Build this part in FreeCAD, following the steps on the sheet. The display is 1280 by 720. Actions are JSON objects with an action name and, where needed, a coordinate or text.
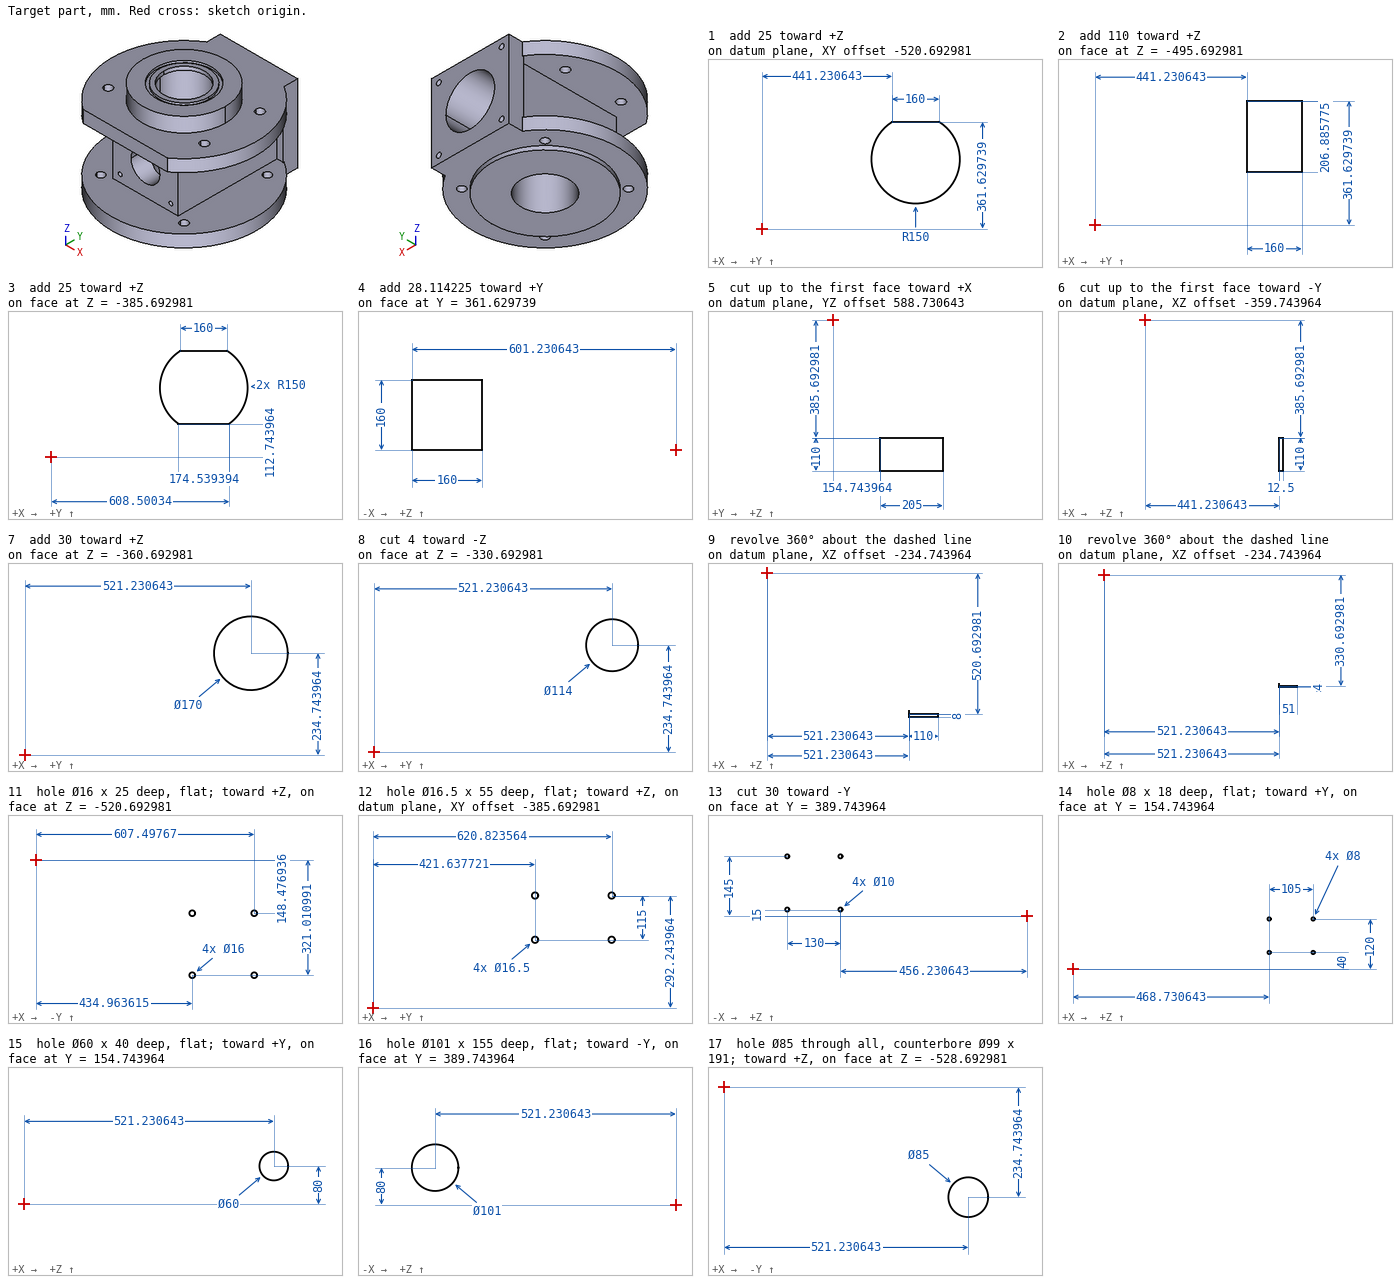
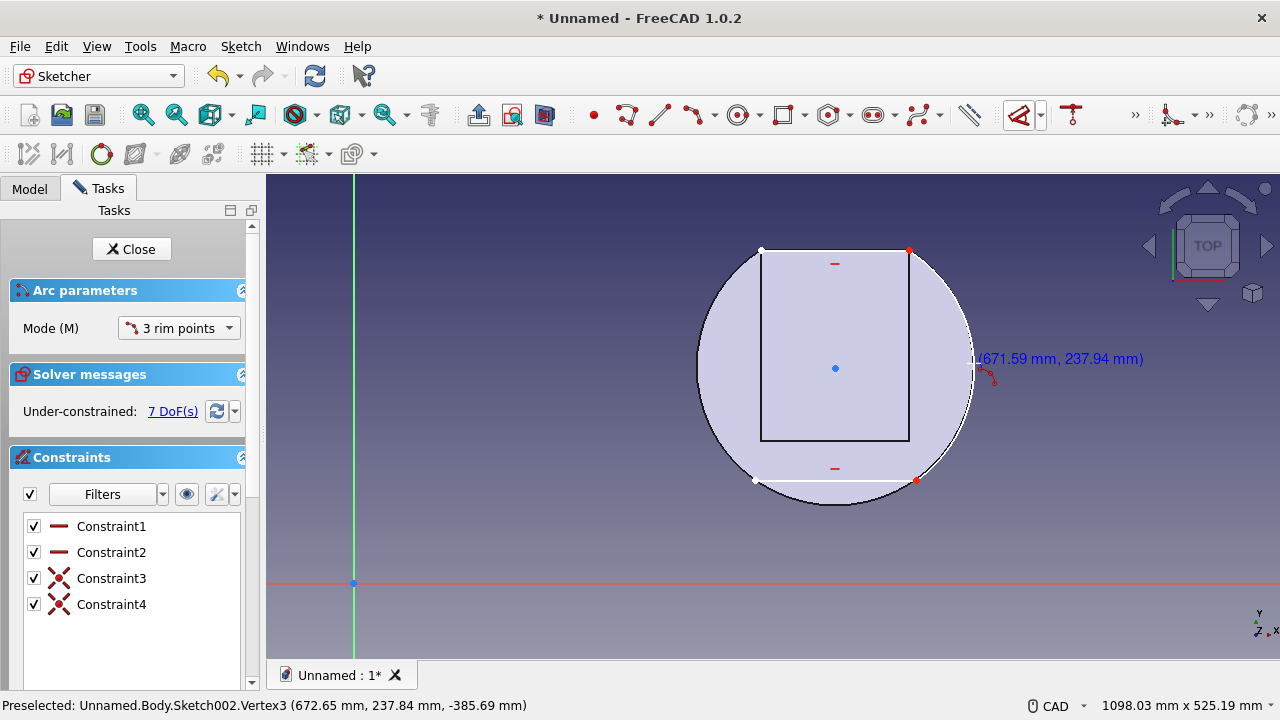
{"action": "left_click", "coordinate": [761, 251]}
{"action": "left_click", "coordinate": [755, 481]}
{"action": "left_click", "coordinate": [697, 363]}
{"action": "key", "text": "Escape"}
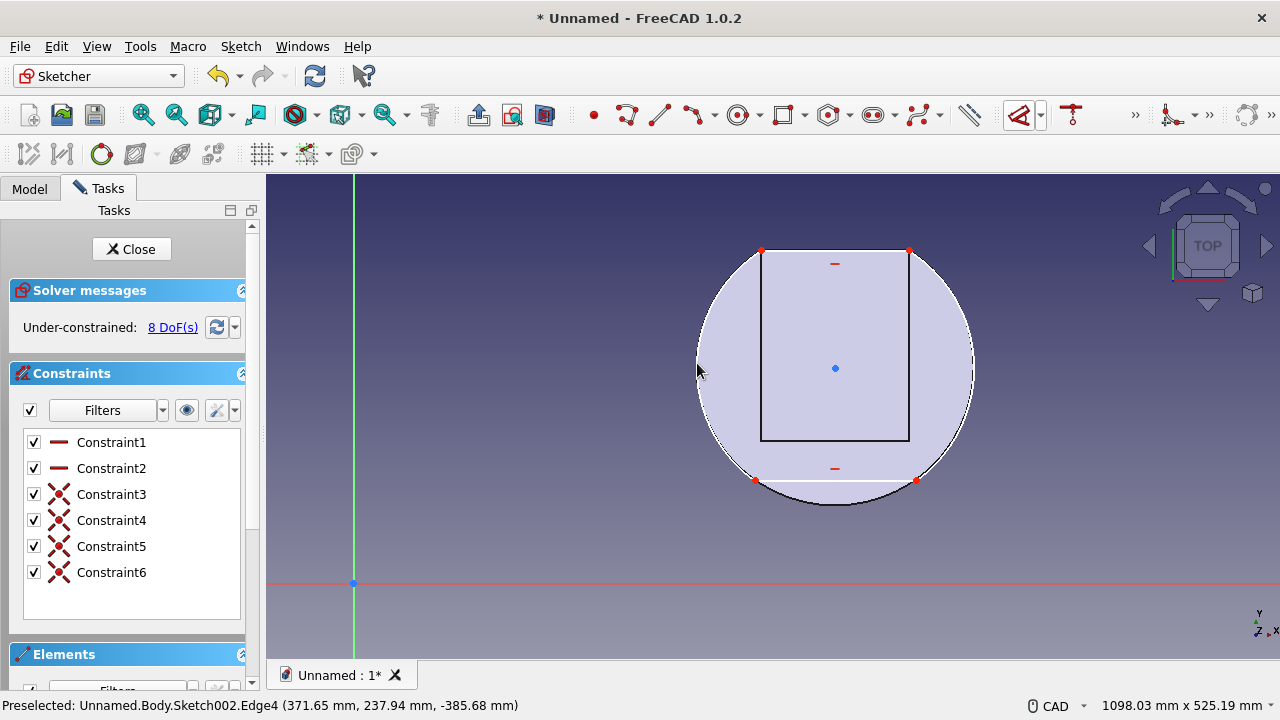
{"action": "left_click", "coordinate": [965, 417]}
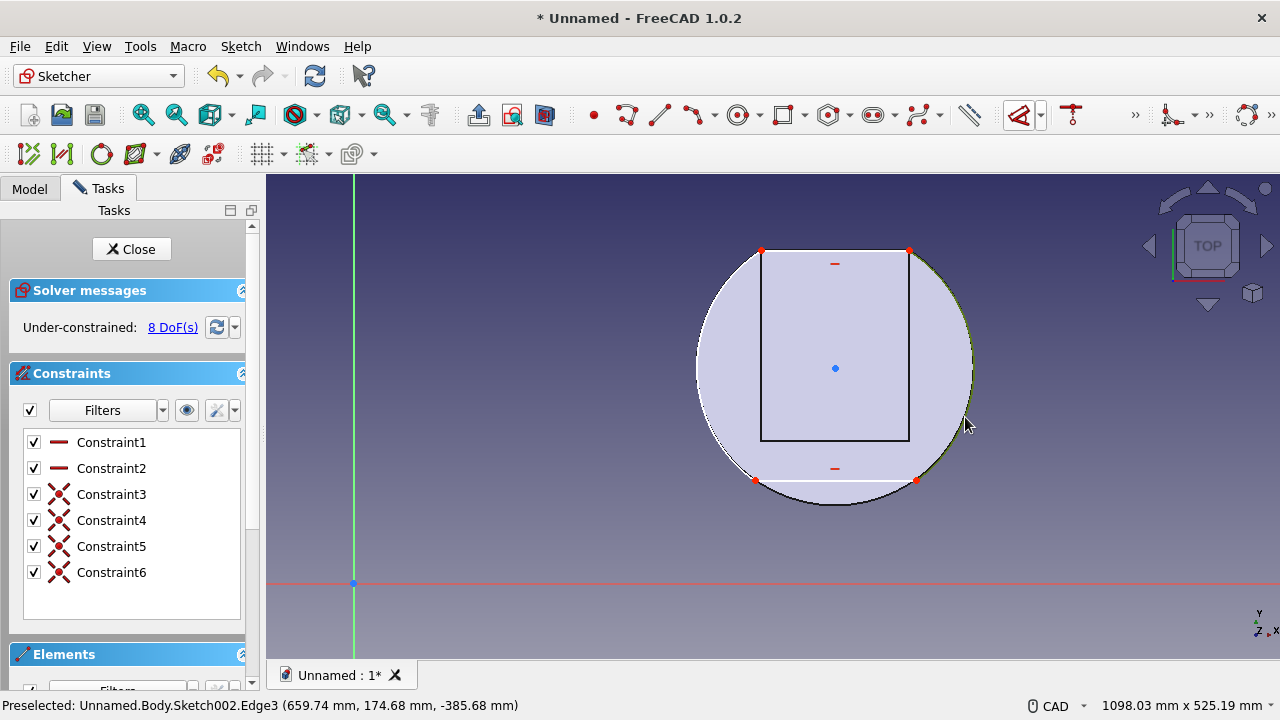
{"action": "left_click", "coordinate": [709, 312]}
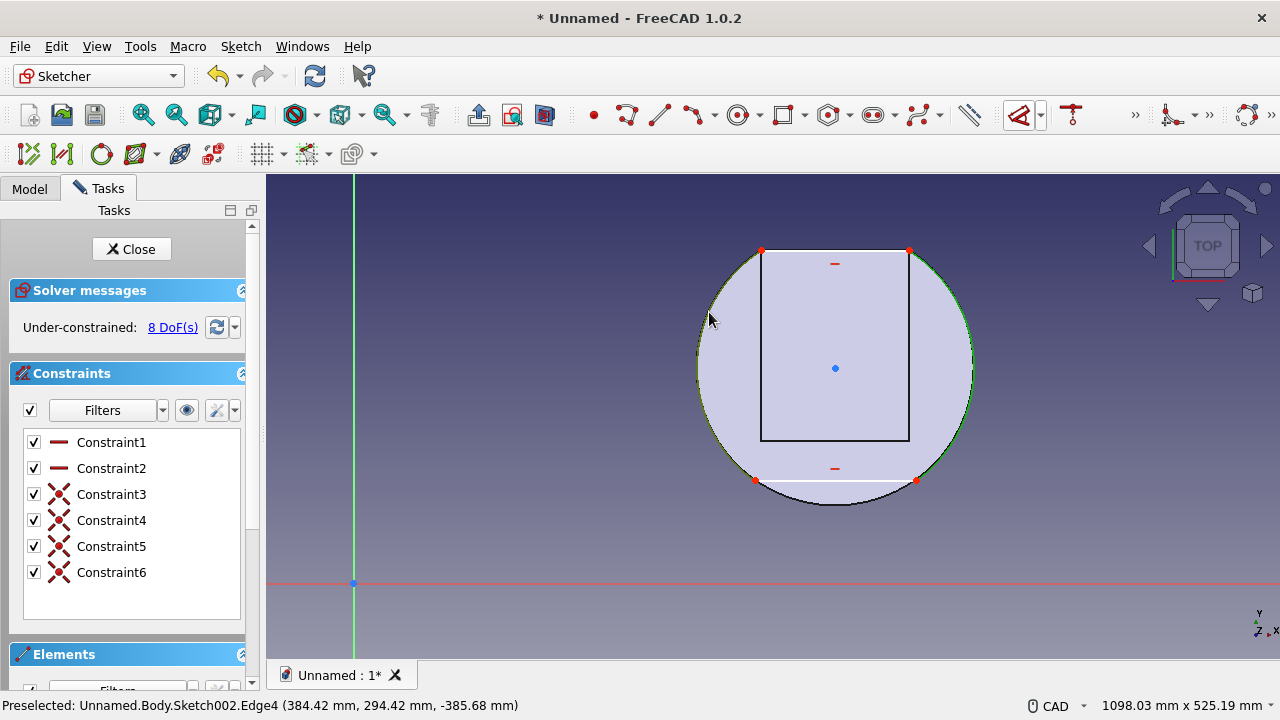
{"action": "left_click", "coordinate": [1071, 116]}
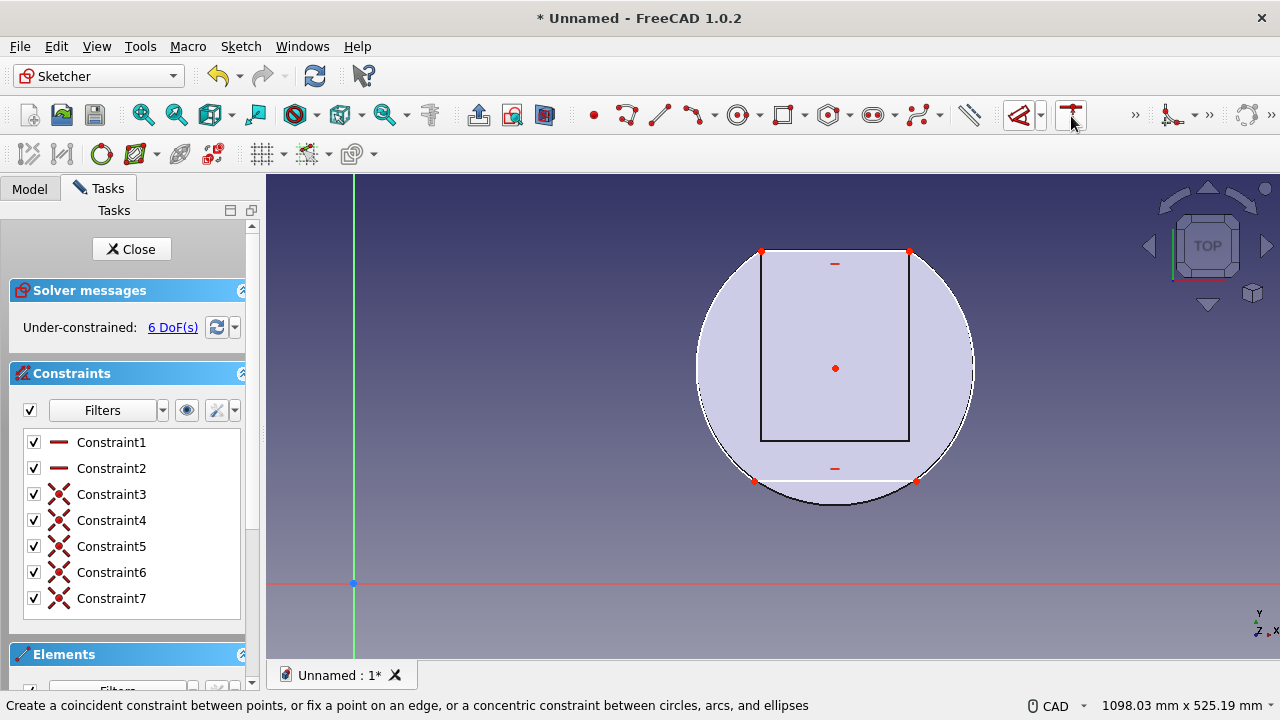
{"action": "left_click", "coordinate": [965, 417]}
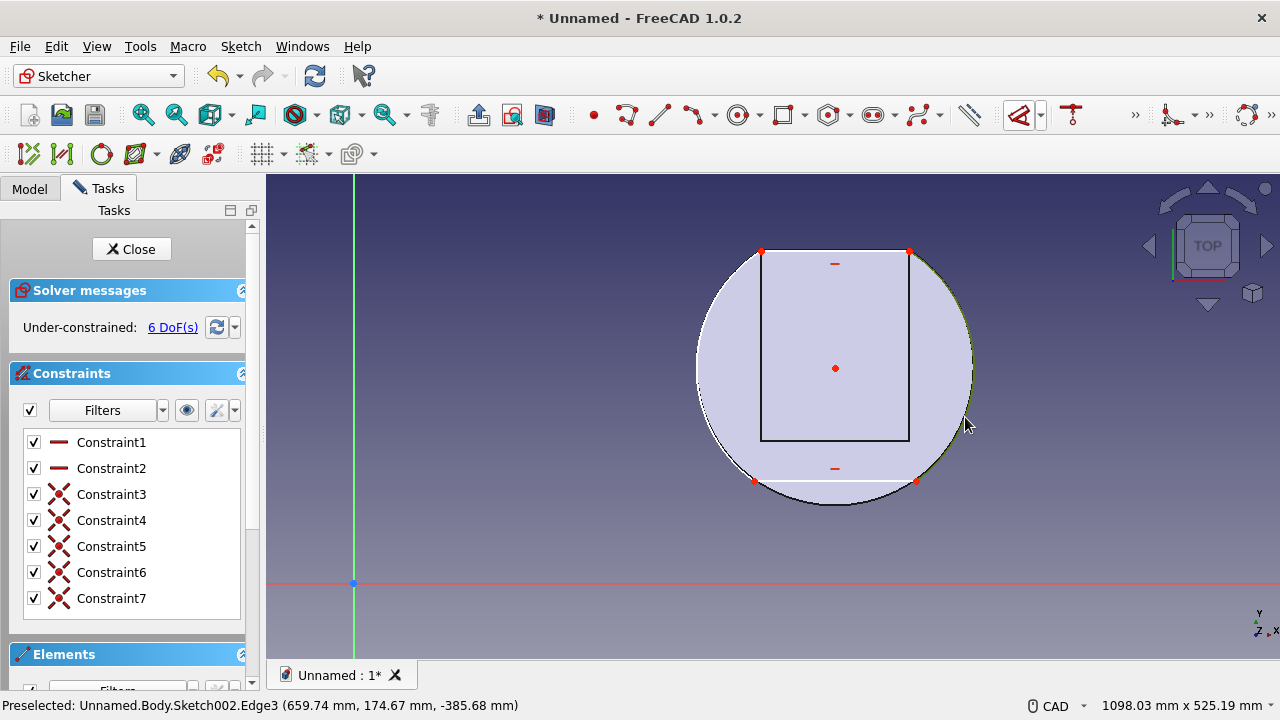
{"action": "left_click", "coordinate": [709, 312]}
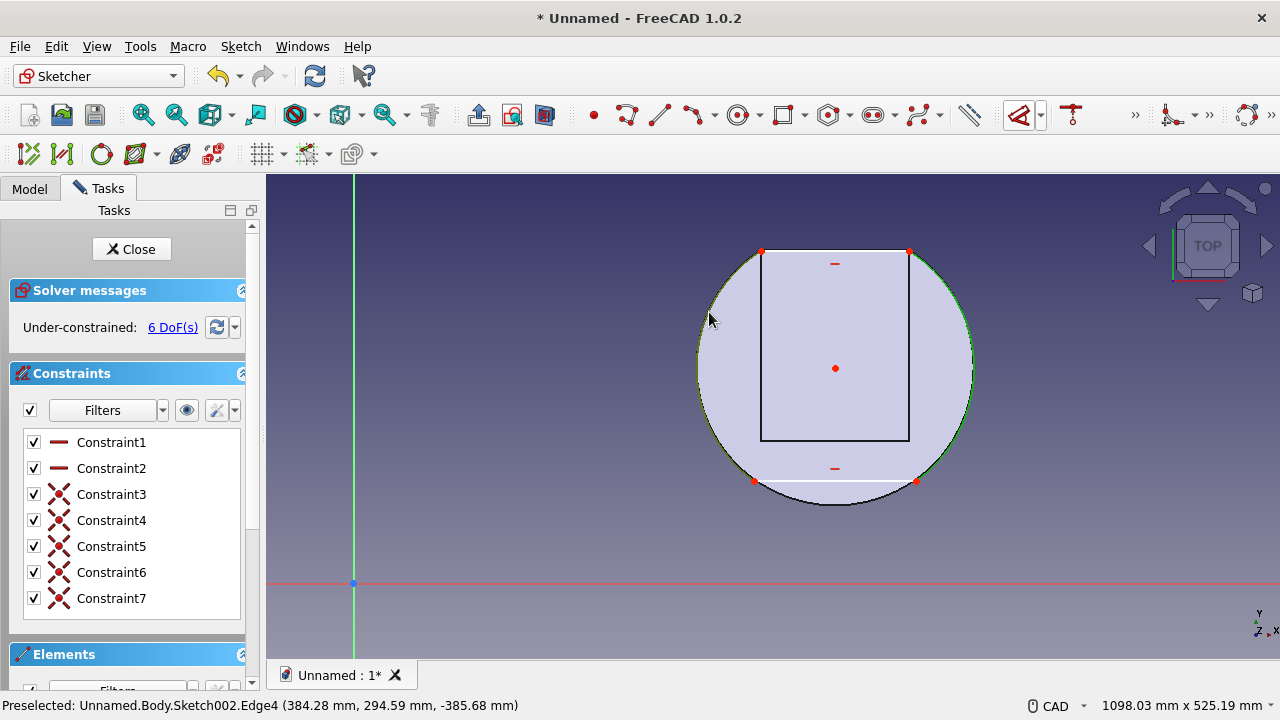
{"action": "key", "text": "e"}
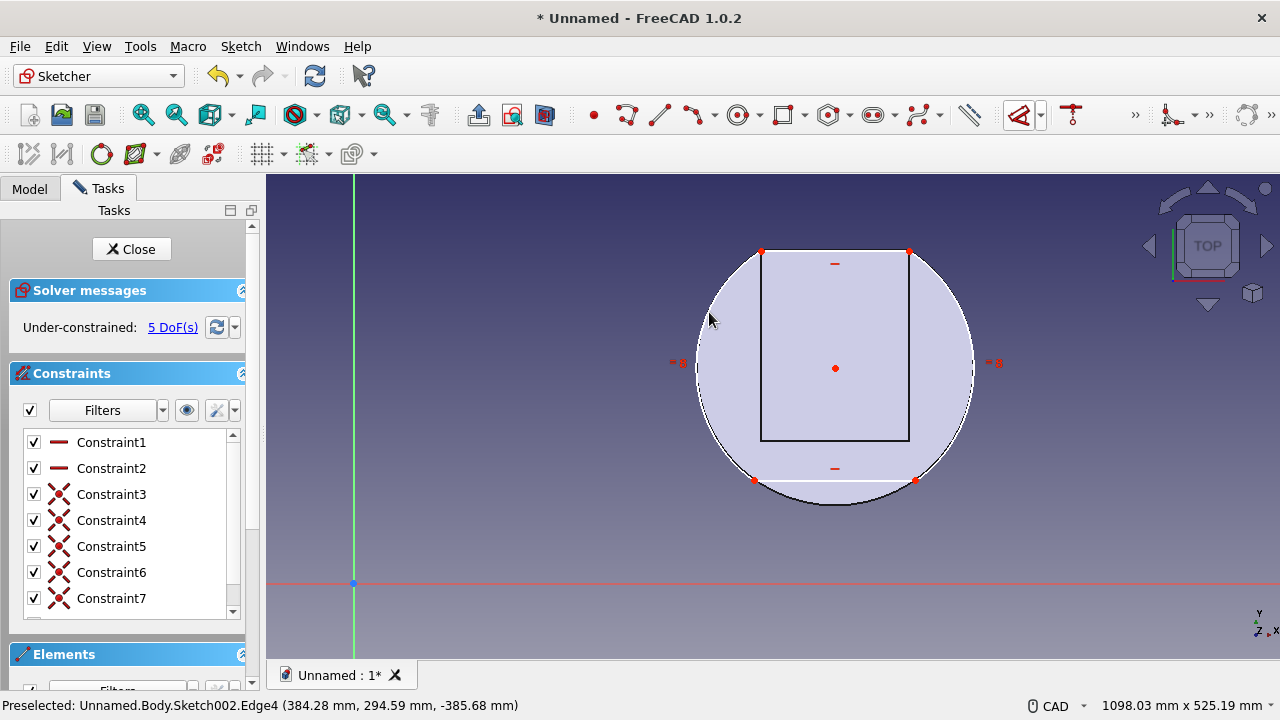
{"action": "left_click", "coordinate": [965, 417]}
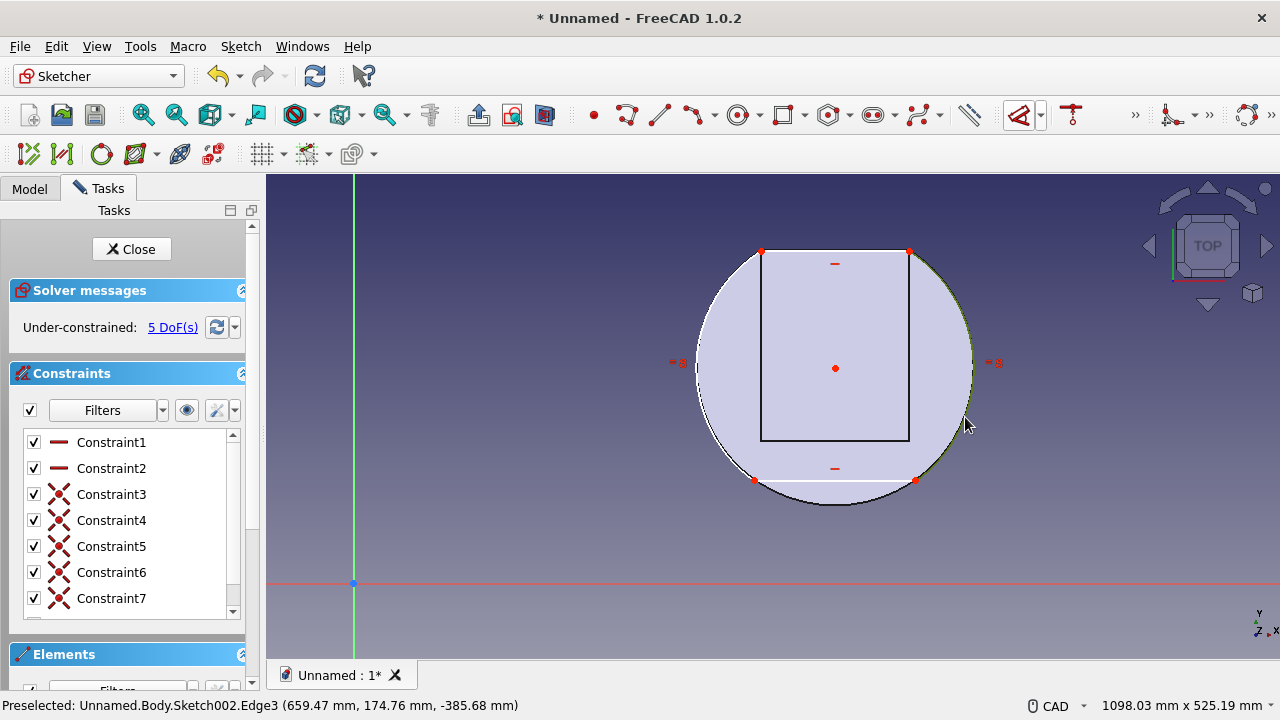
{"action": "left_click", "coordinate": [1040, 116]}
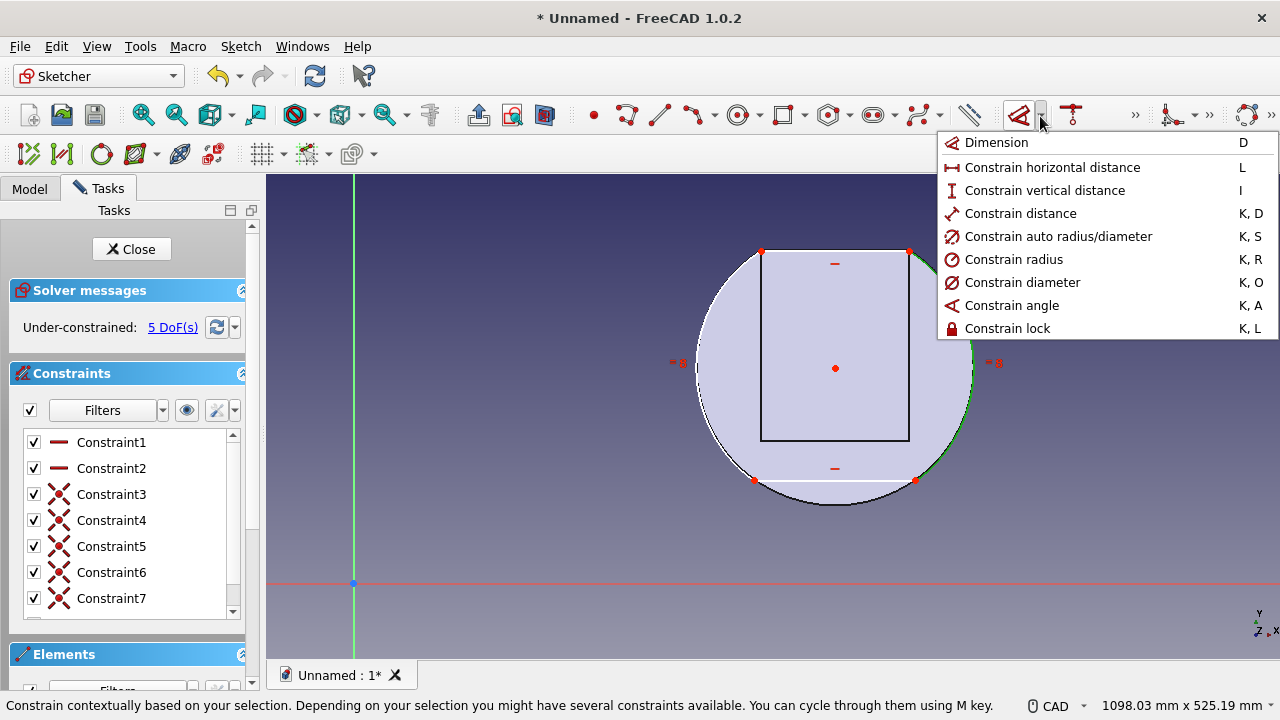
{"action": "left_click", "coordinate": [1108, 260]}